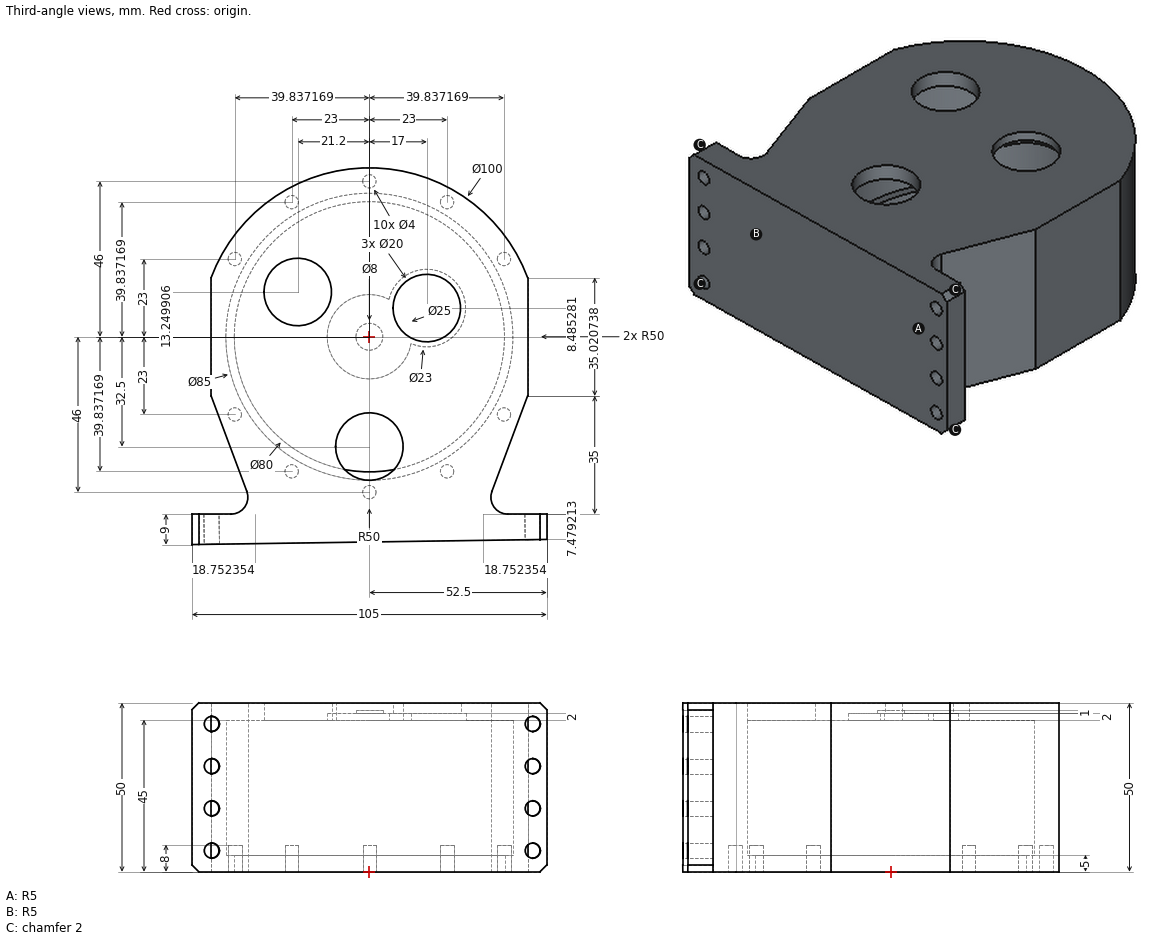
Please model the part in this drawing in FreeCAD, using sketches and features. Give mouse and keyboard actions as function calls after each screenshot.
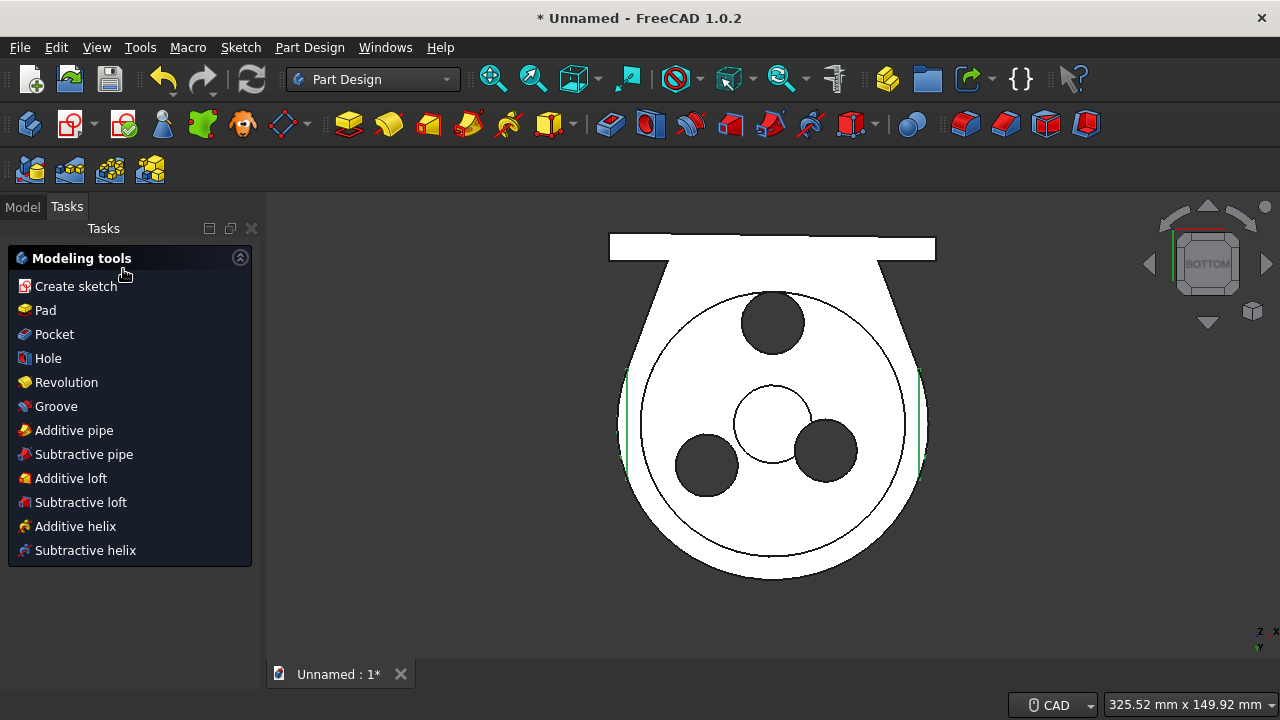
click(612, 124)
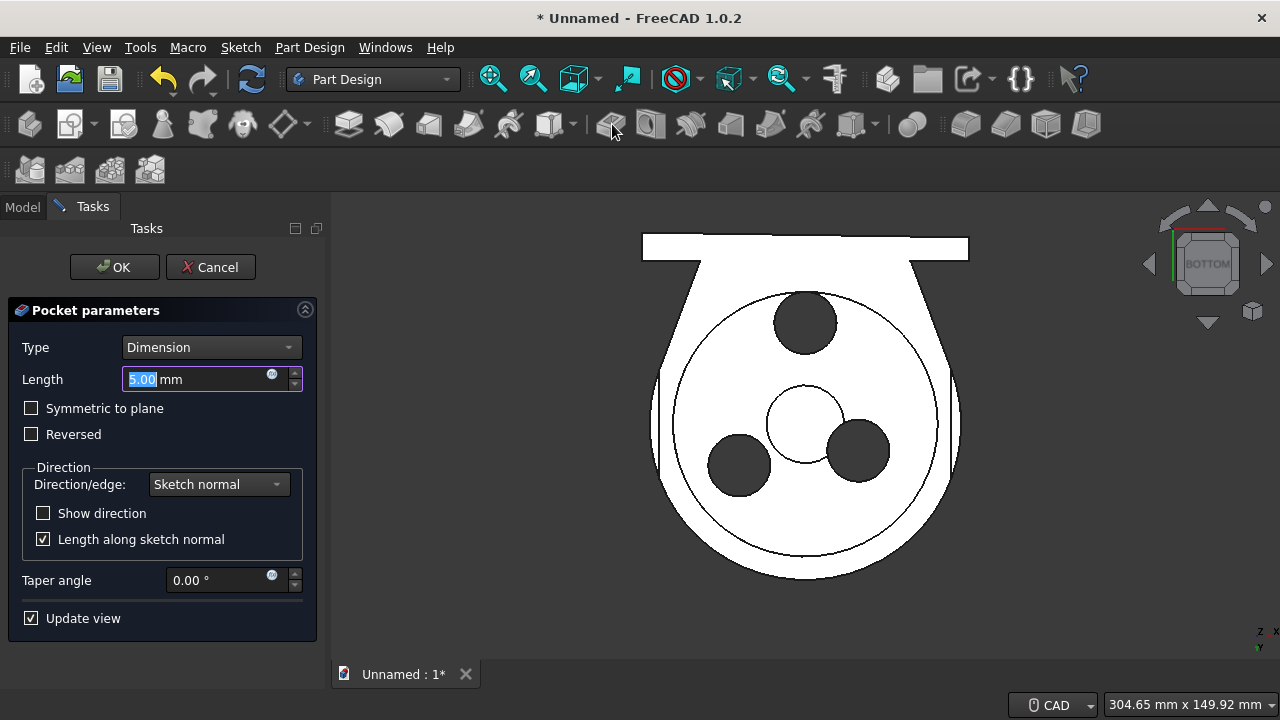
click(212, 348)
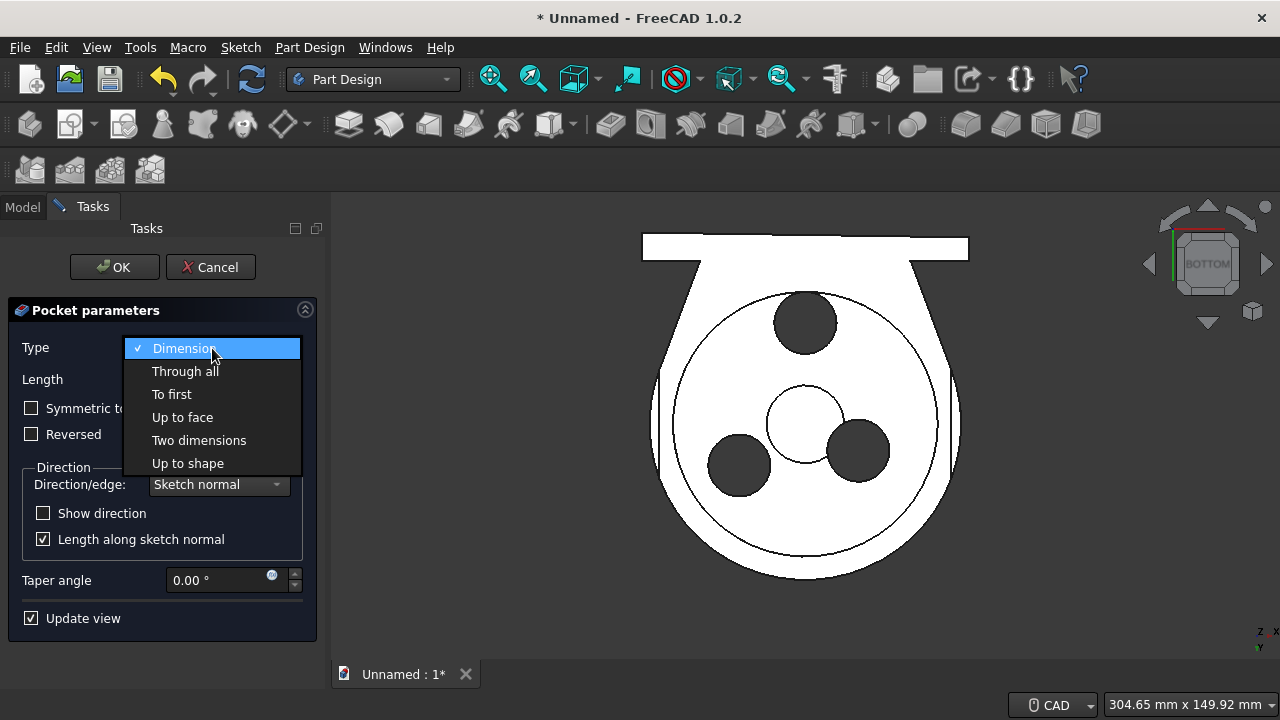
click(212, 372)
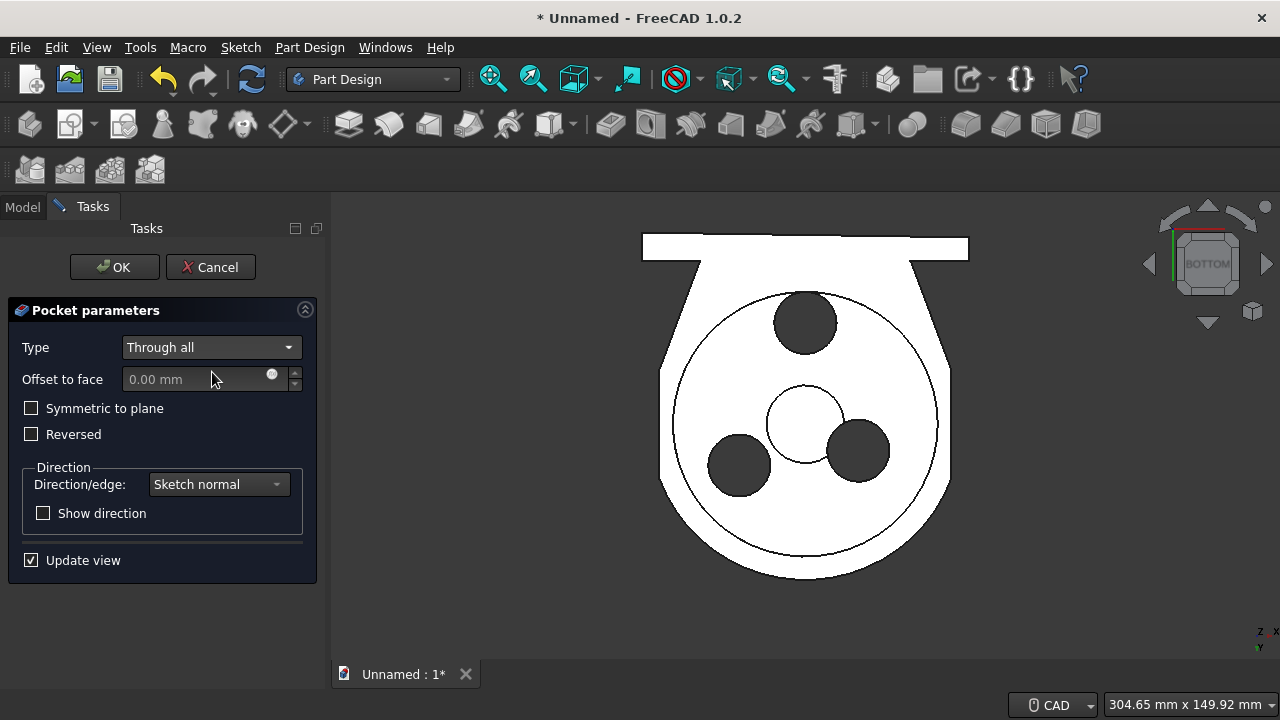
click(115, 267)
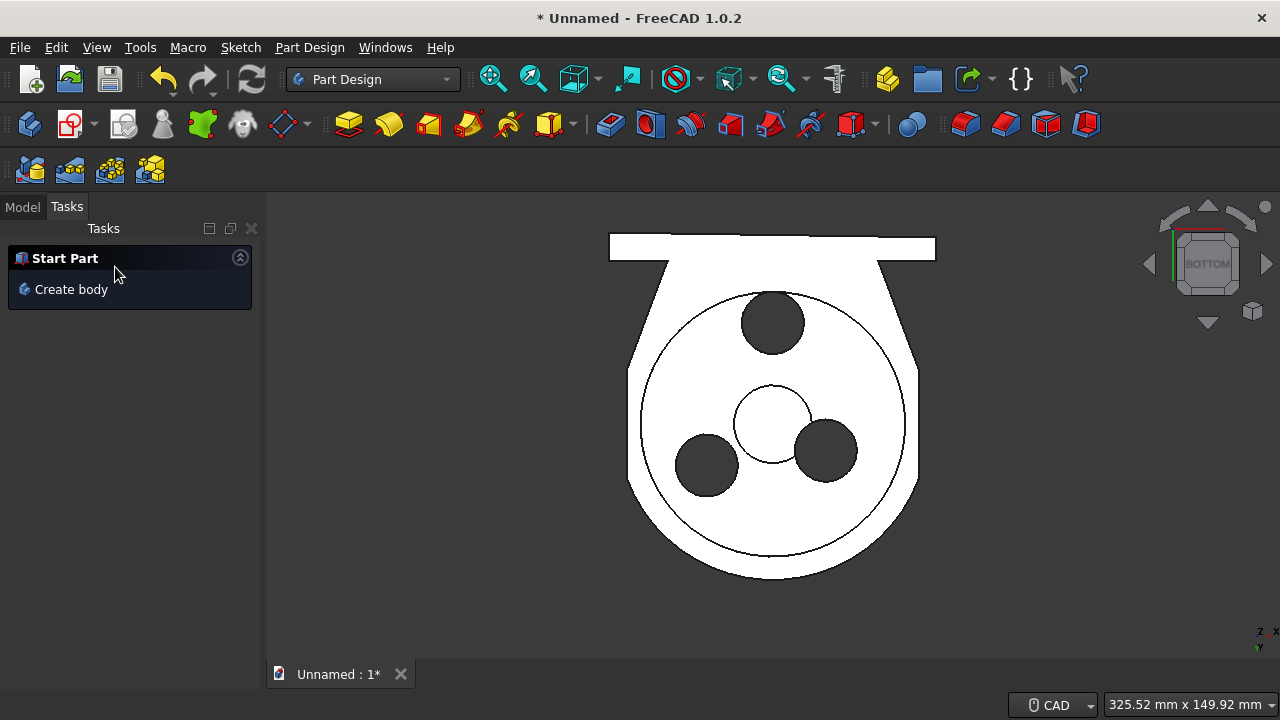
key(0)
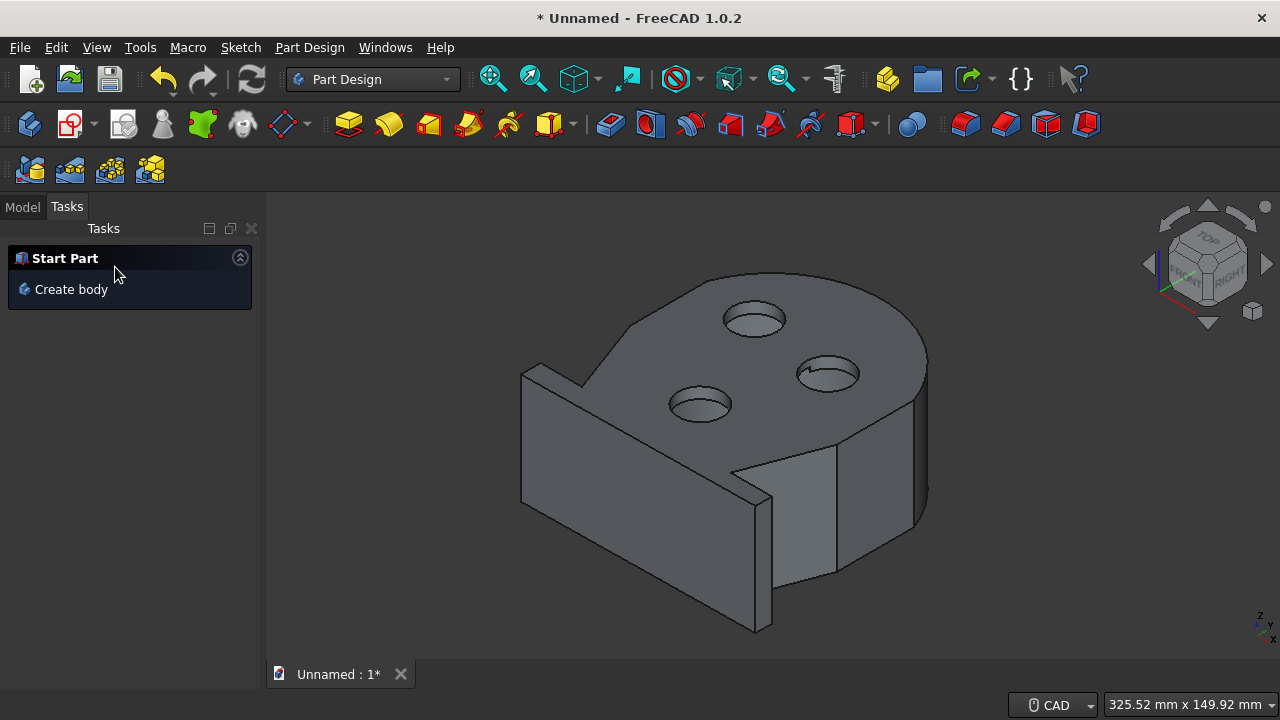
click(672, 522)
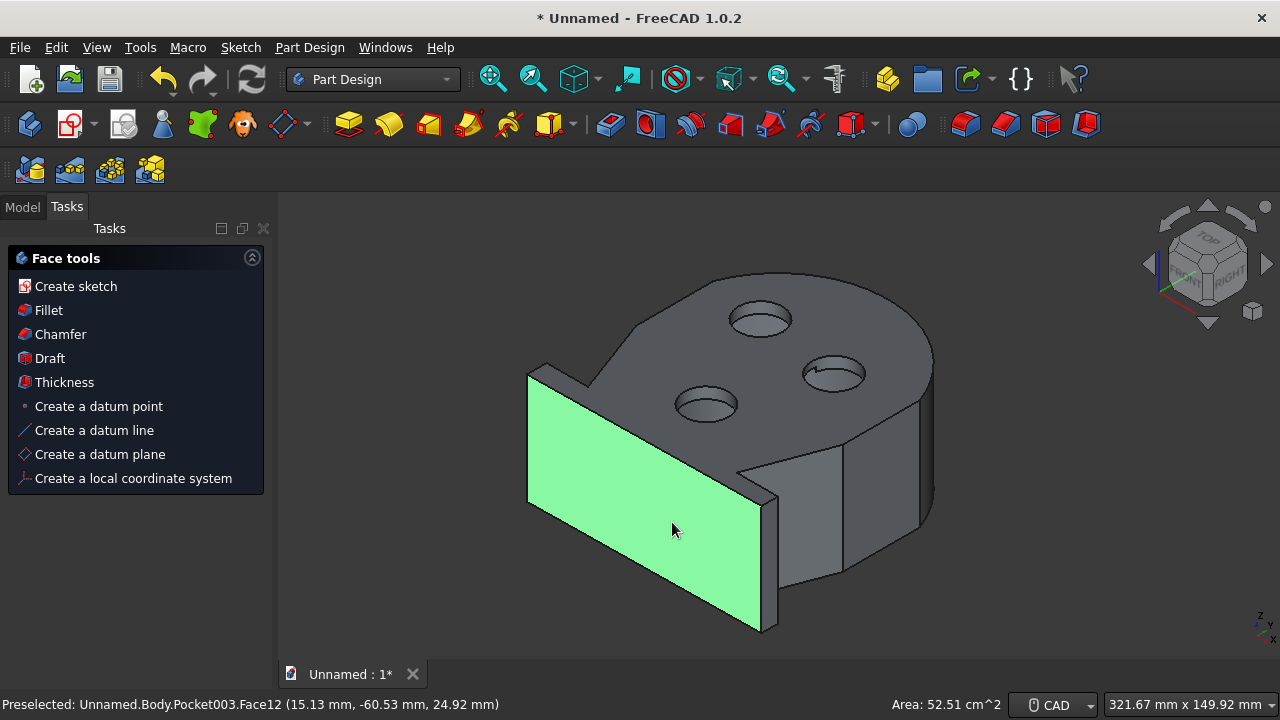
click(70, 124)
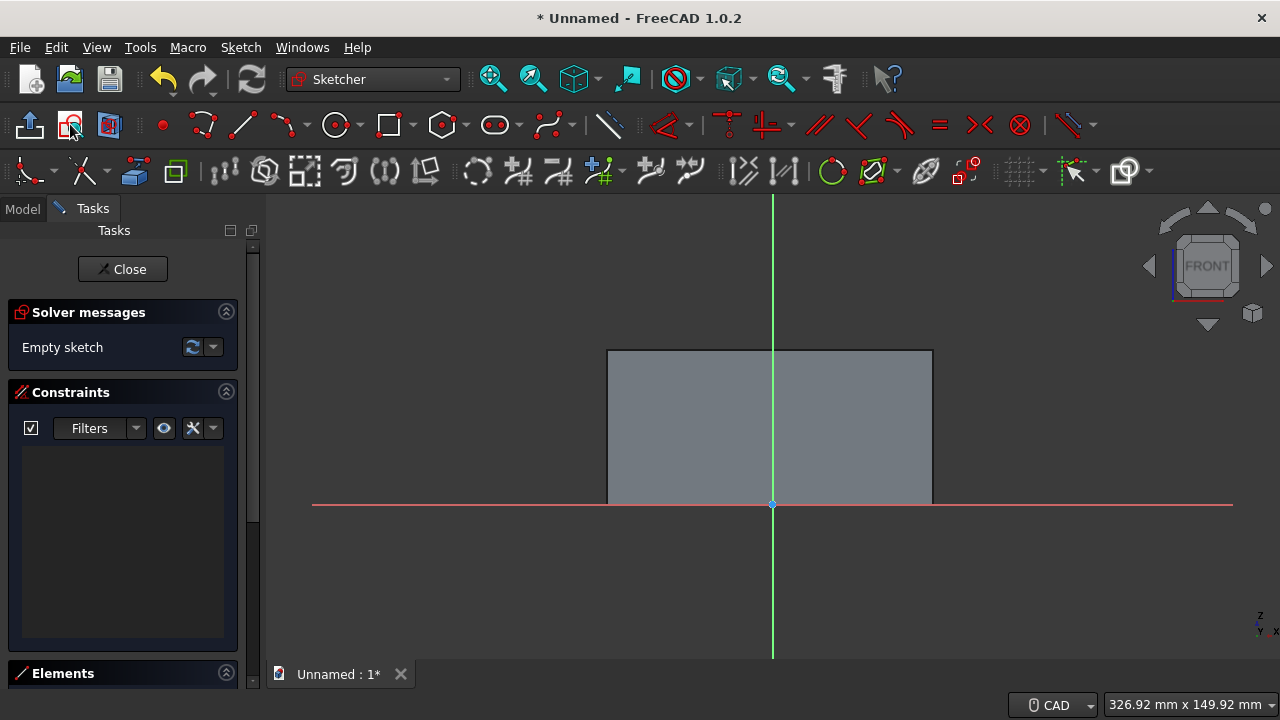
key(q)
key(s)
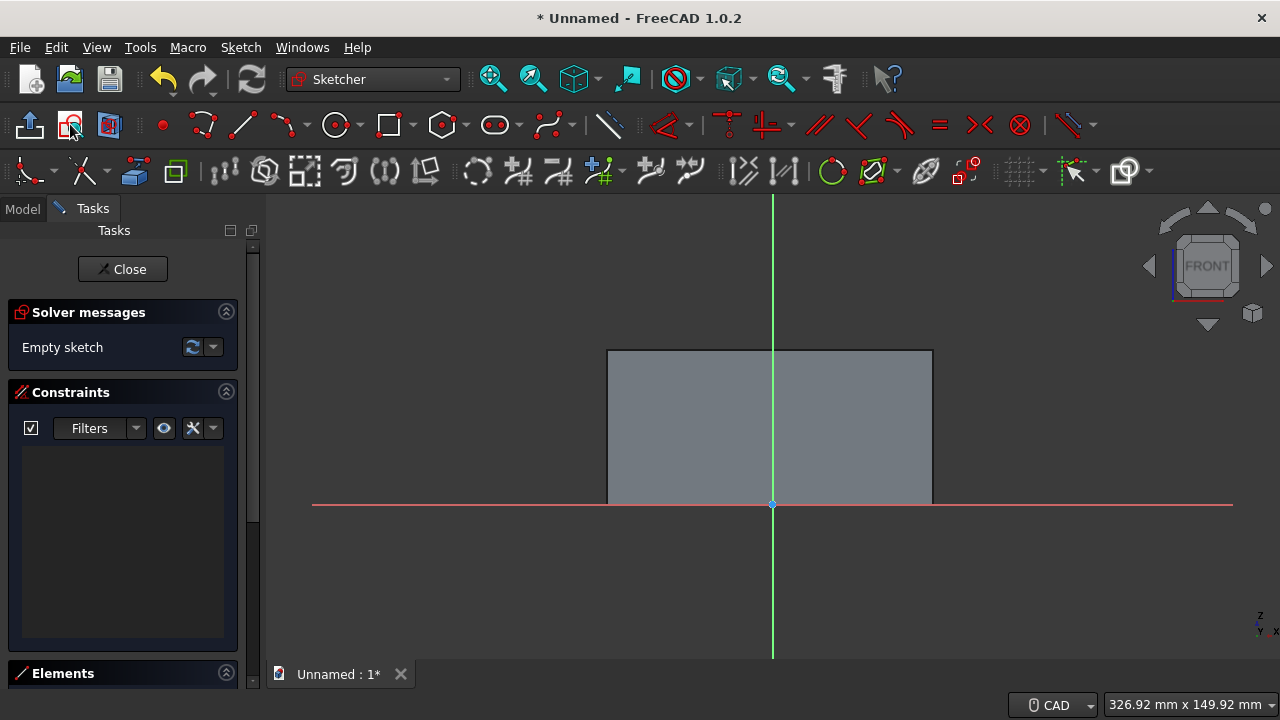
scroll(856, 442, up, 3)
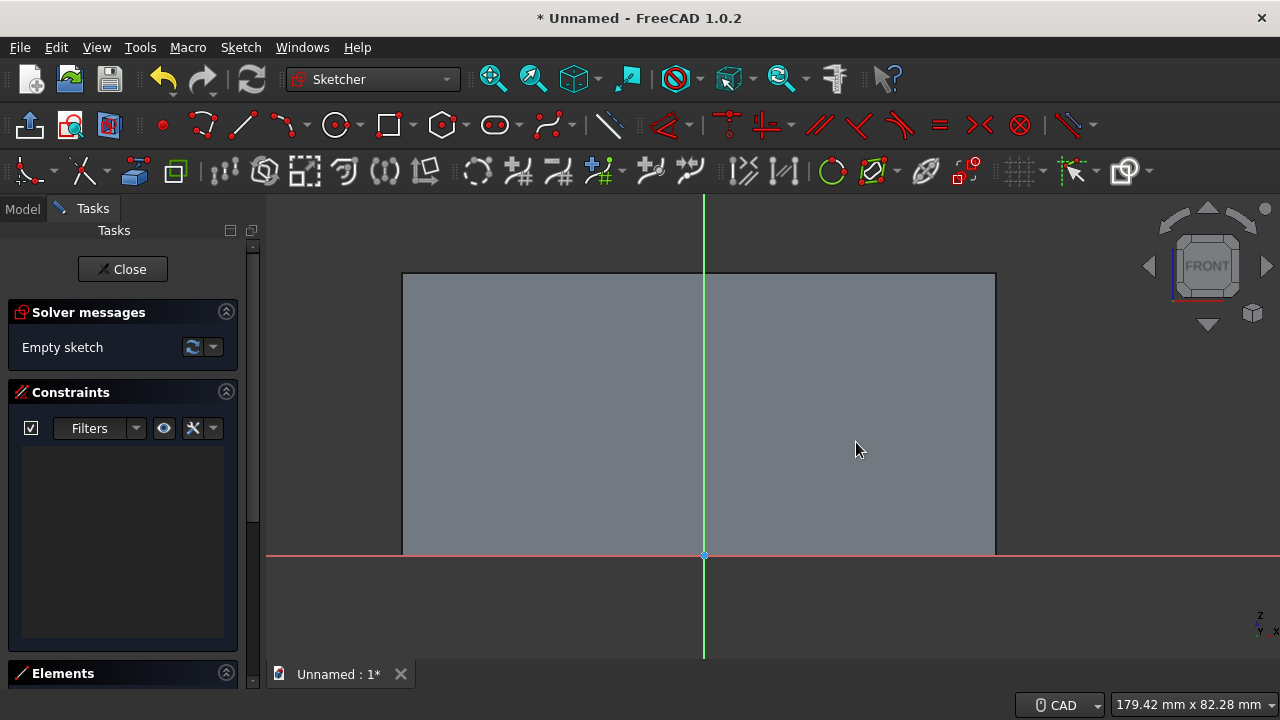
click(336, 126)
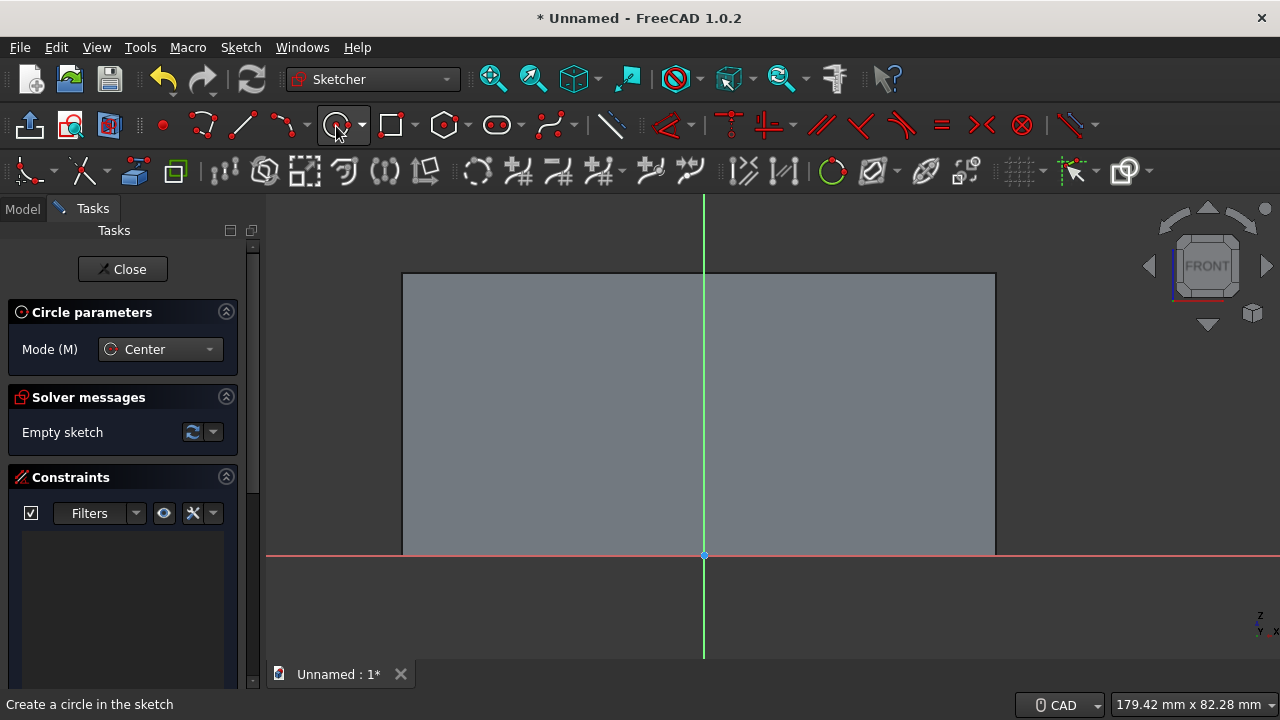
scroll(436, 309, up, 3)